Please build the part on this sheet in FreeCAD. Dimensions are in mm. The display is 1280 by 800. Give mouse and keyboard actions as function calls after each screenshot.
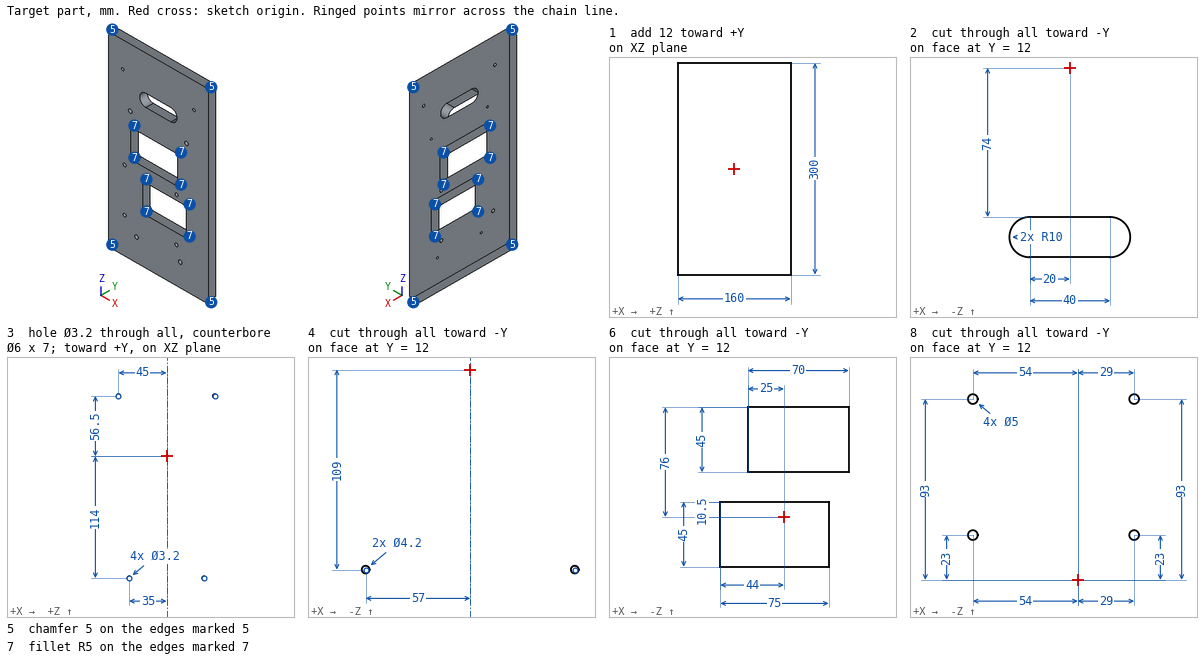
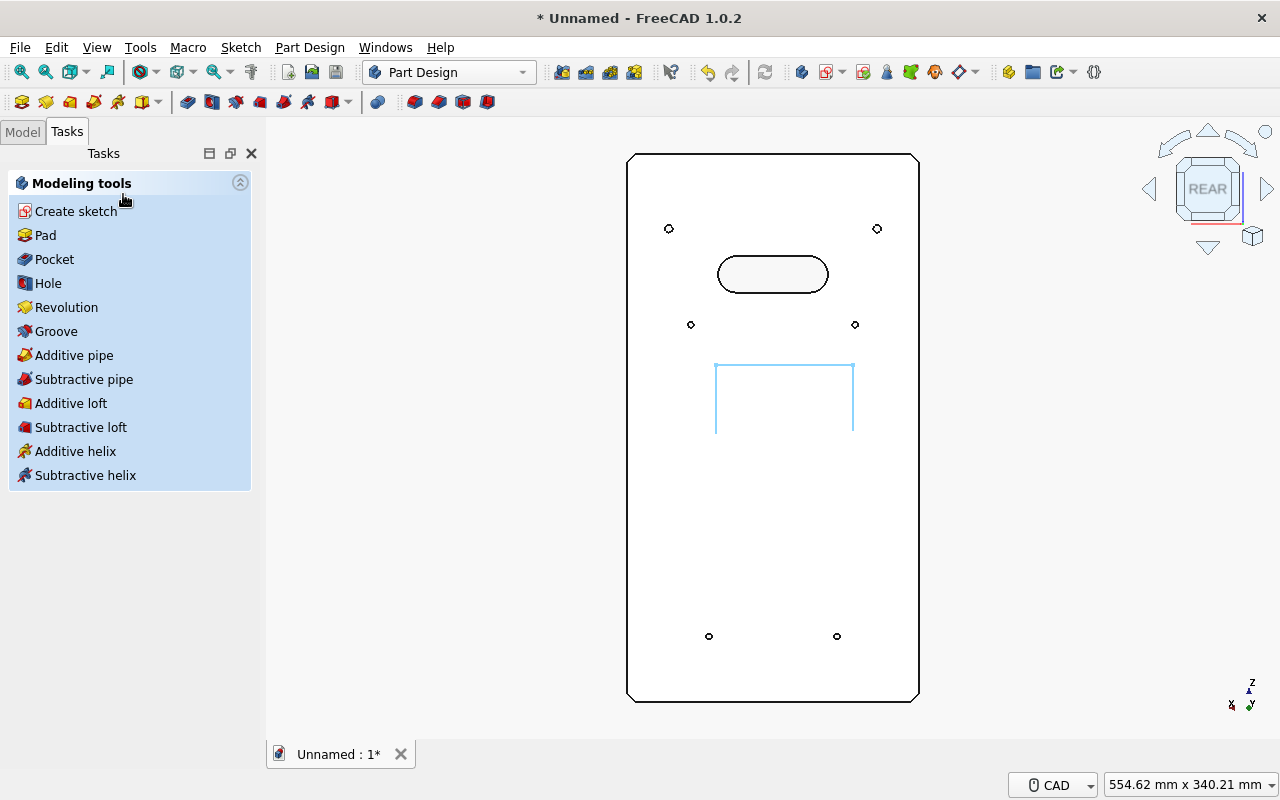
click(188, 102)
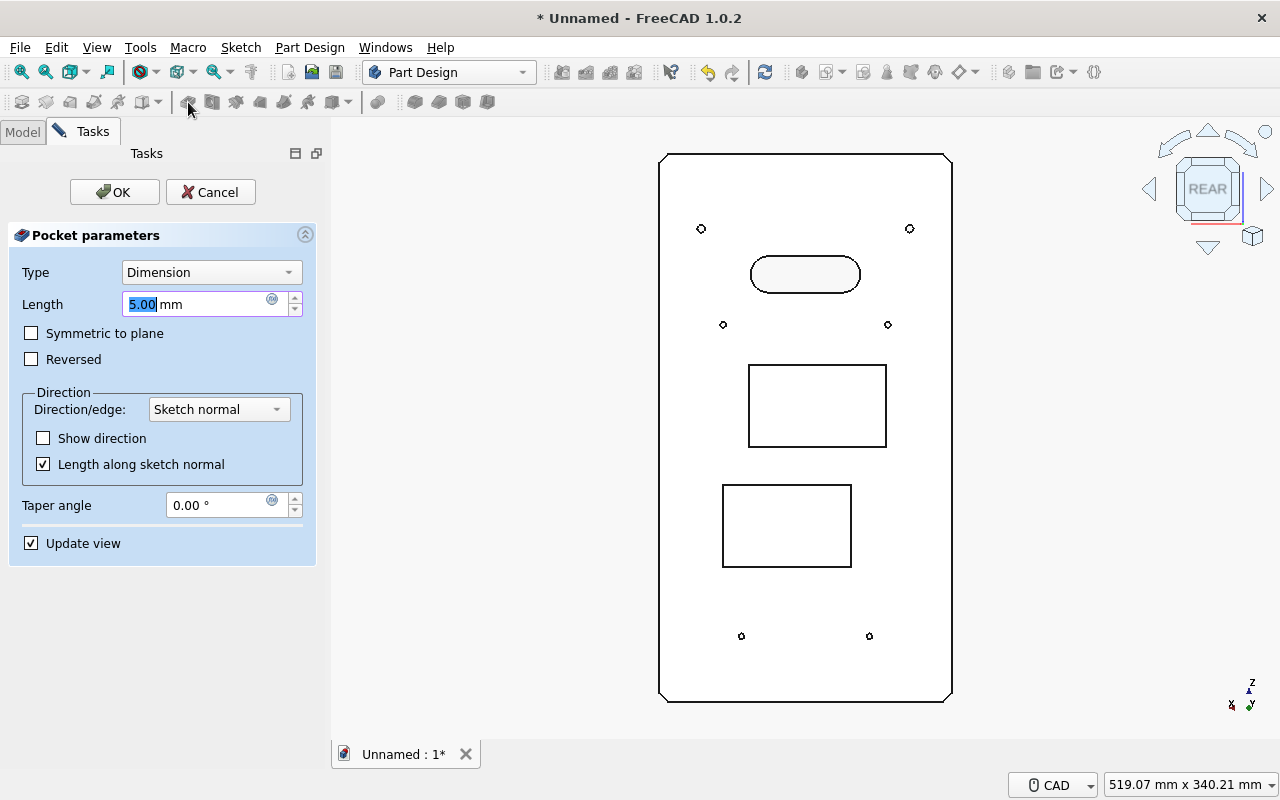
click(212, 272)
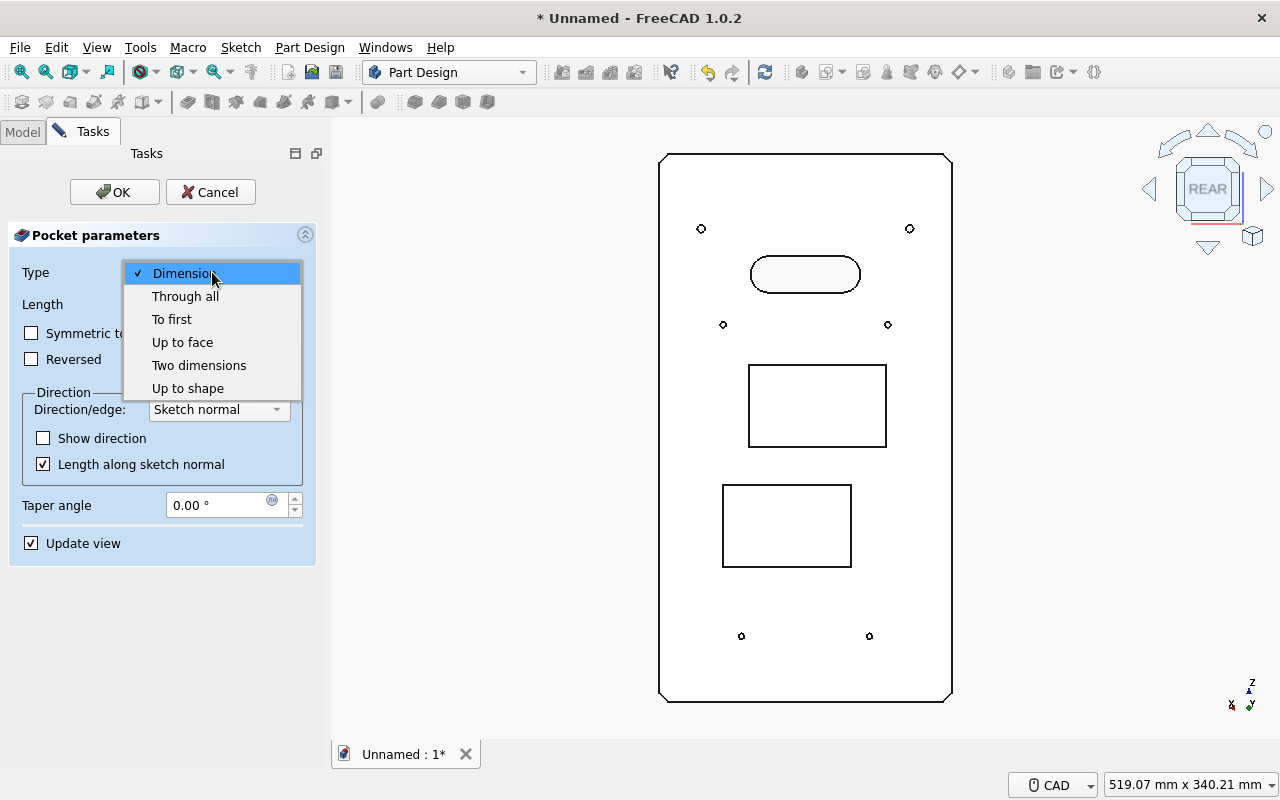
click(212, 296)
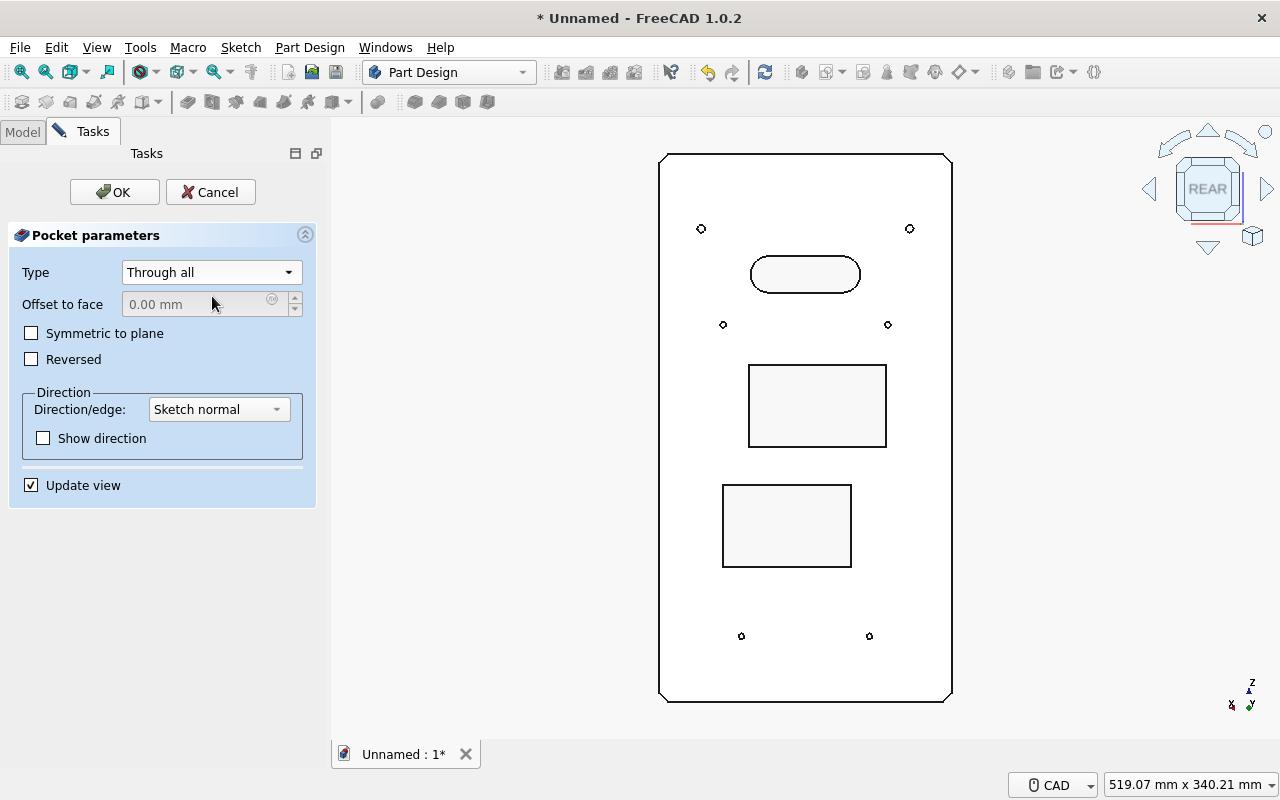
click(115, 192)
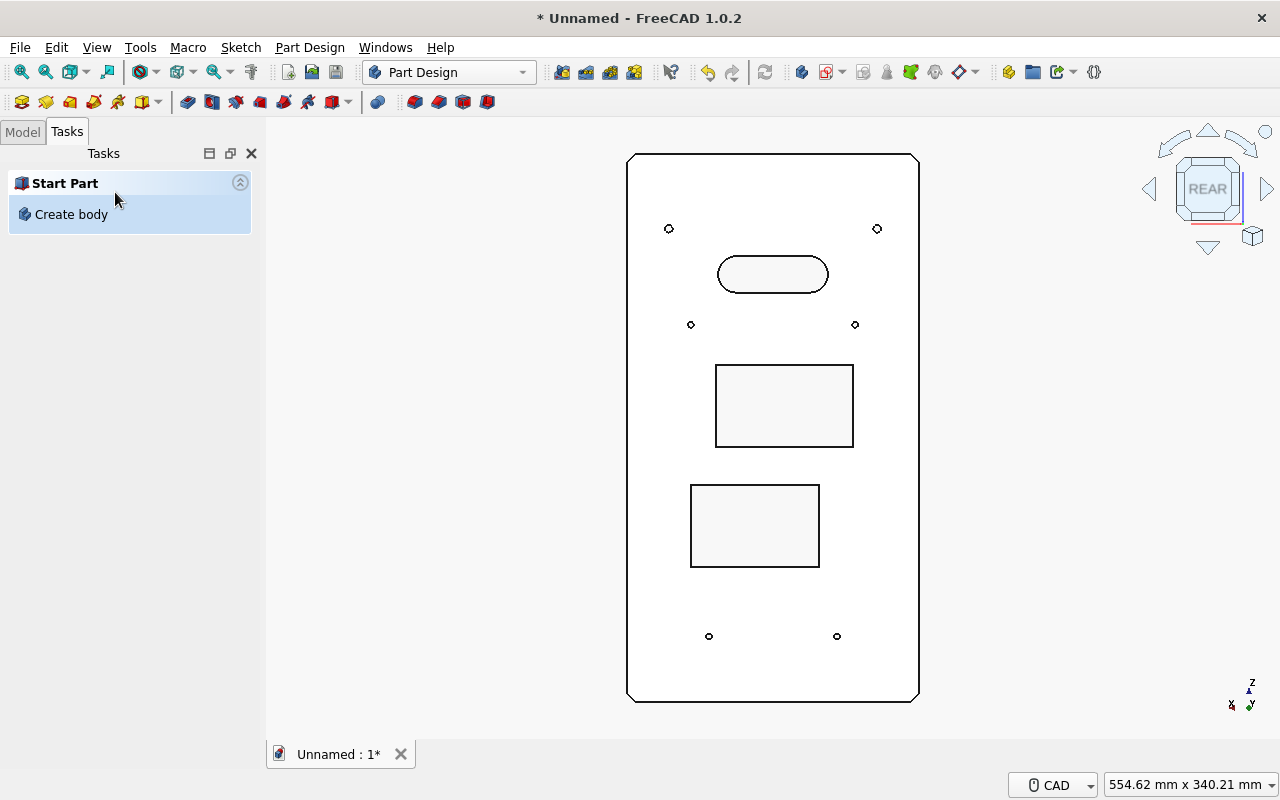
scroll(716, 446, up, 4)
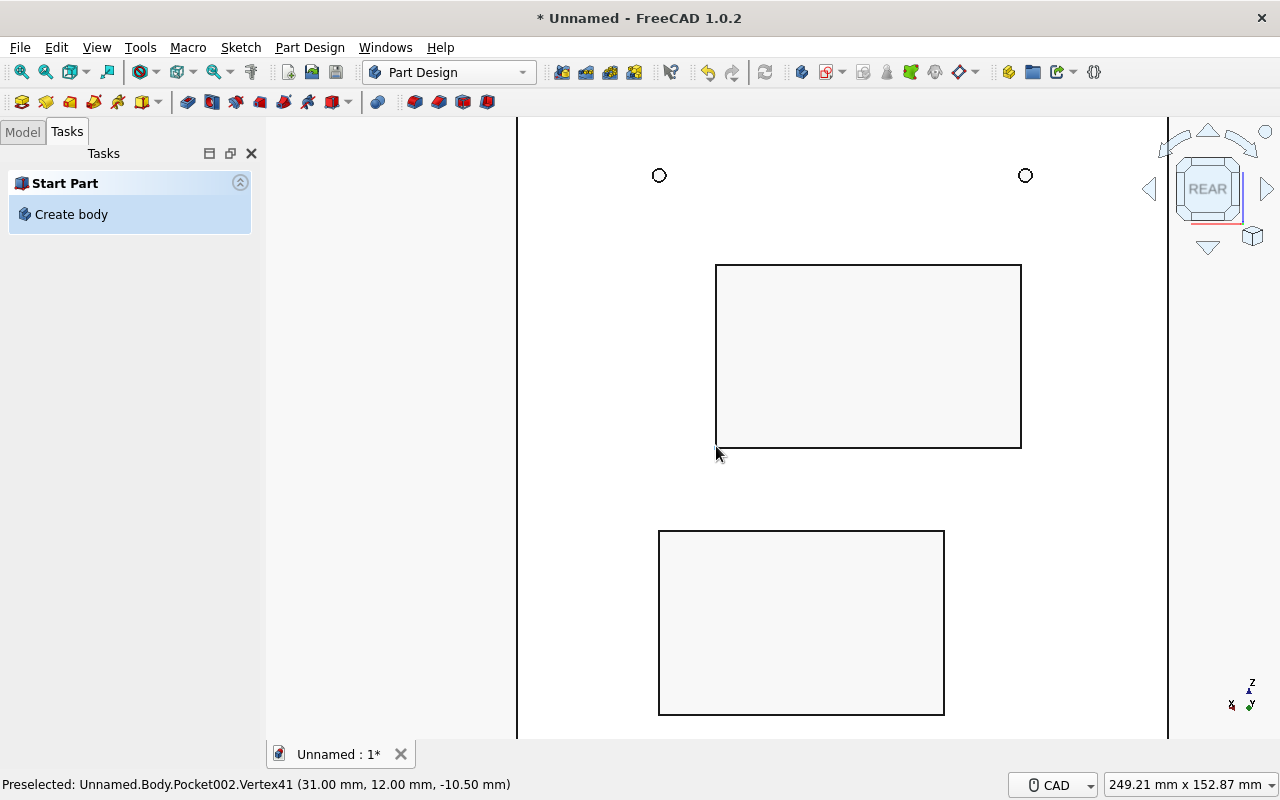
click(22, 72)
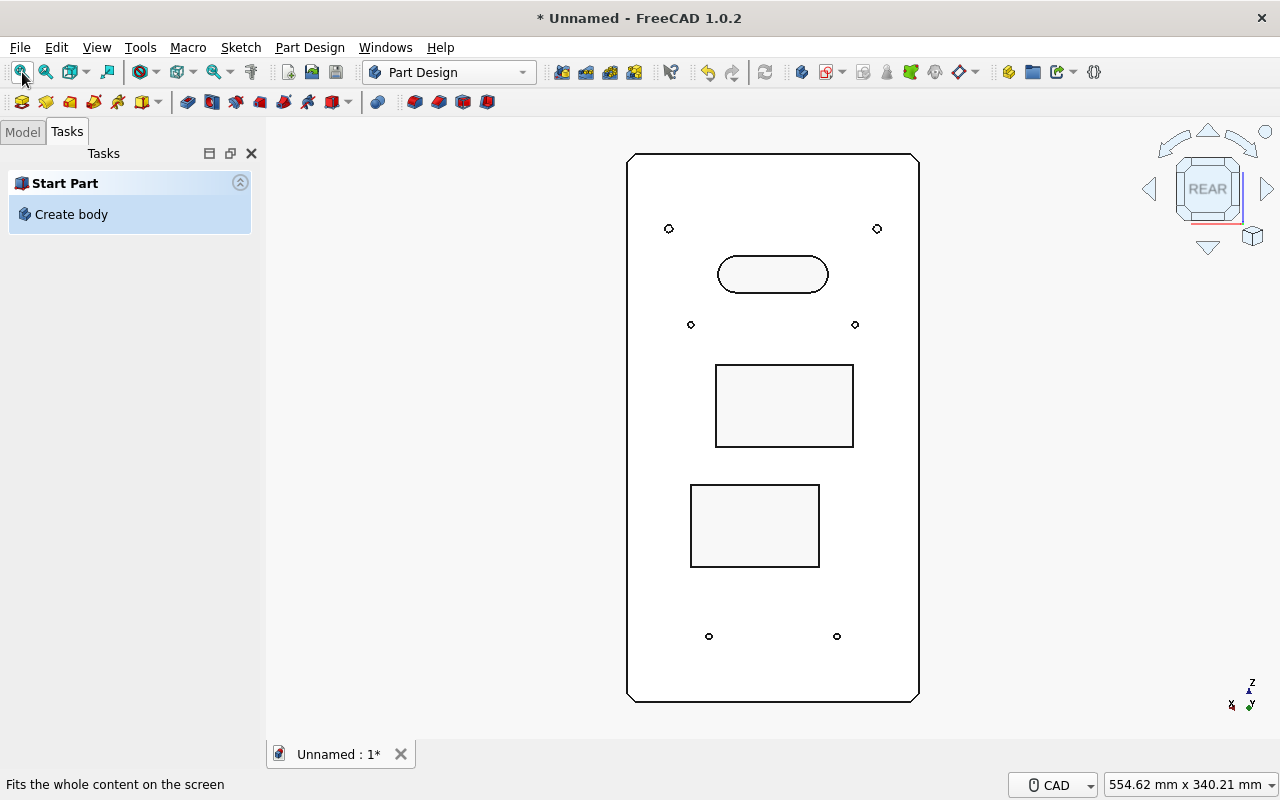
key(0)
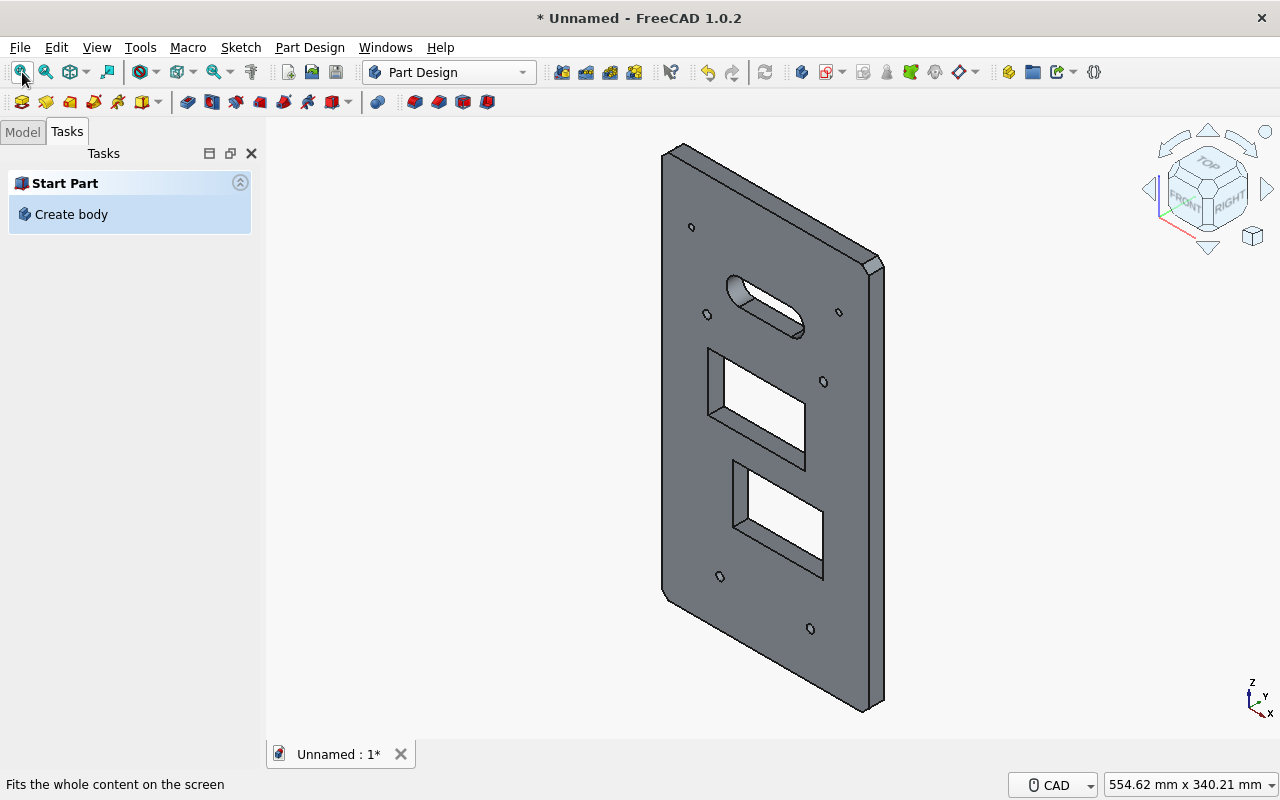
scroll(813, 466, up, 4)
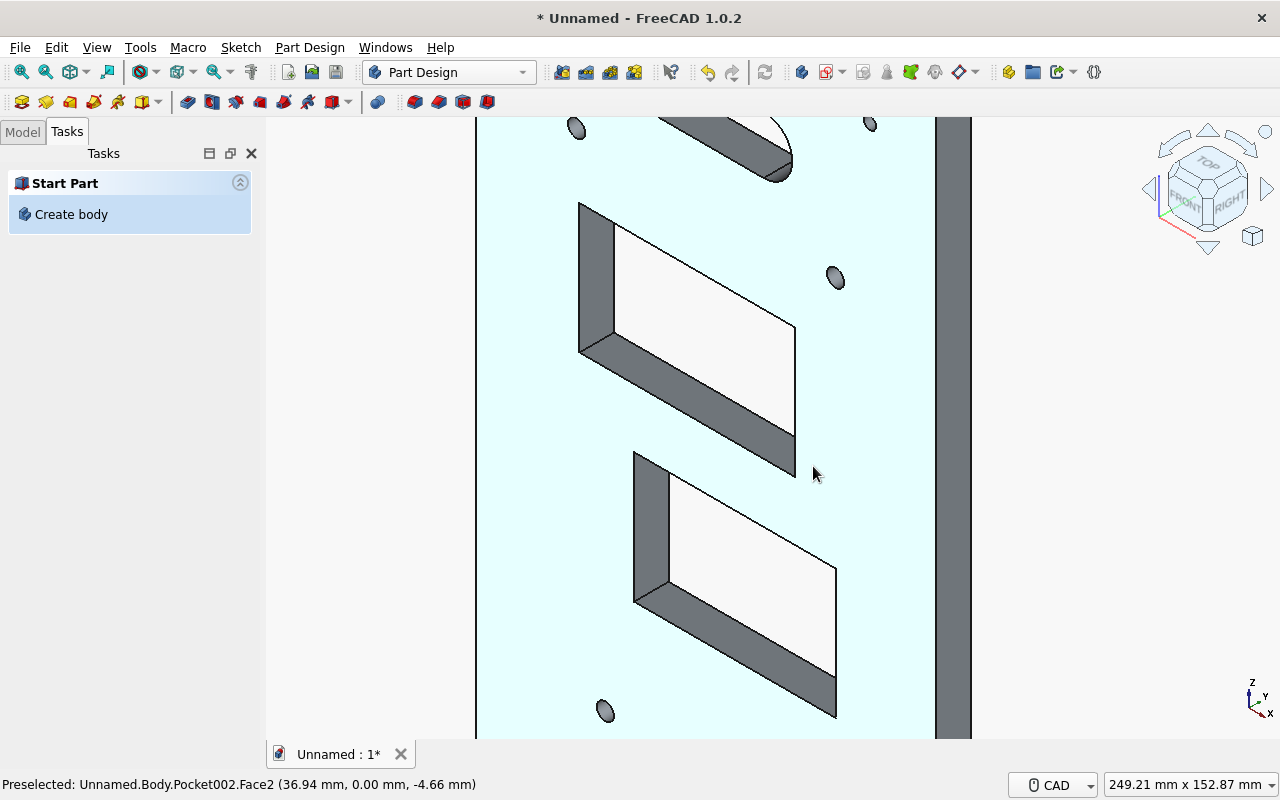
click(22, 72)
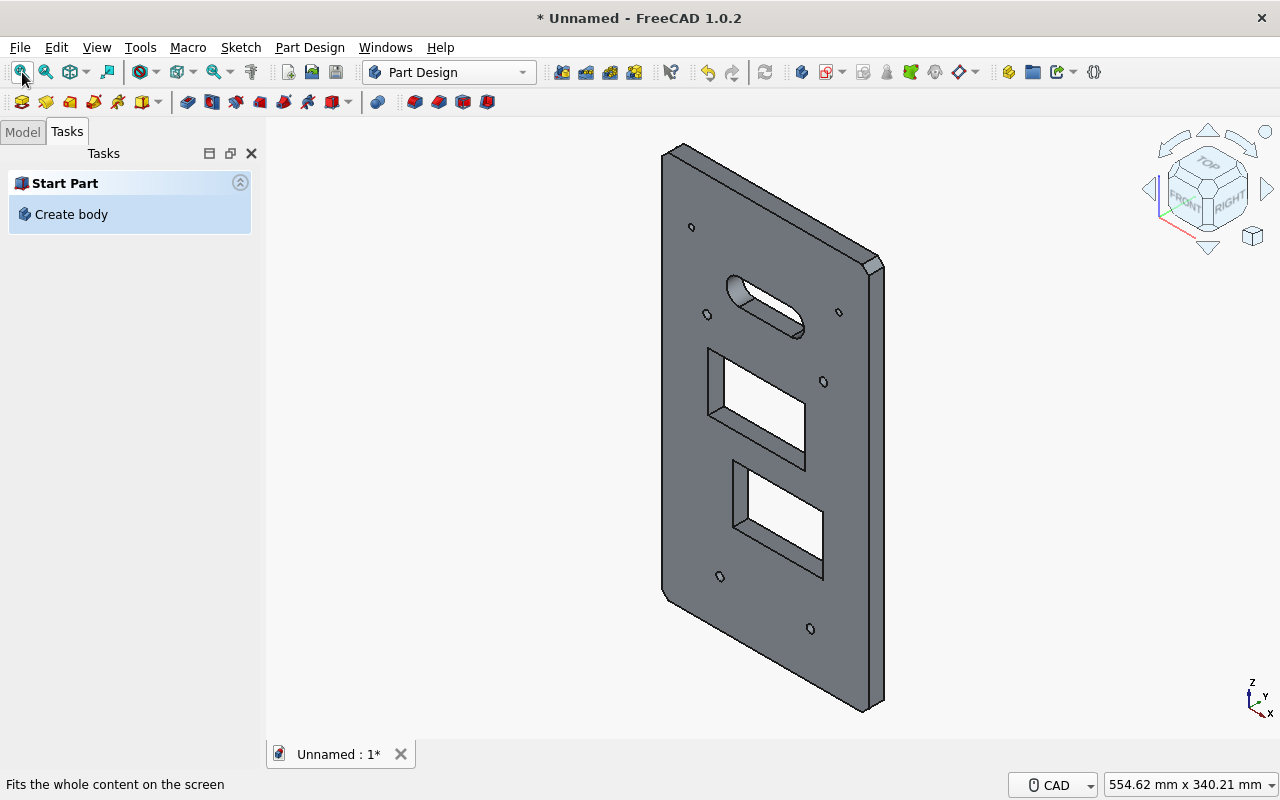
key(2)